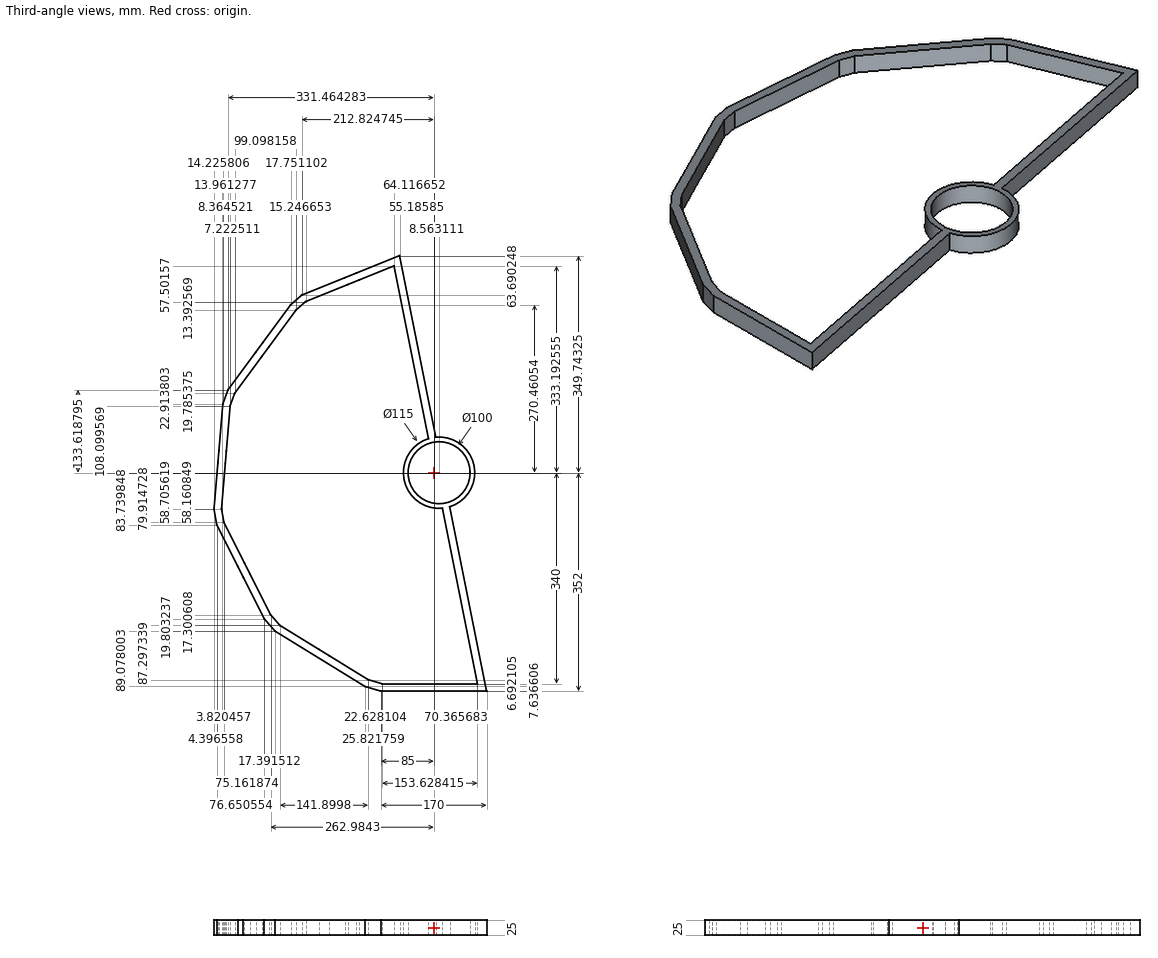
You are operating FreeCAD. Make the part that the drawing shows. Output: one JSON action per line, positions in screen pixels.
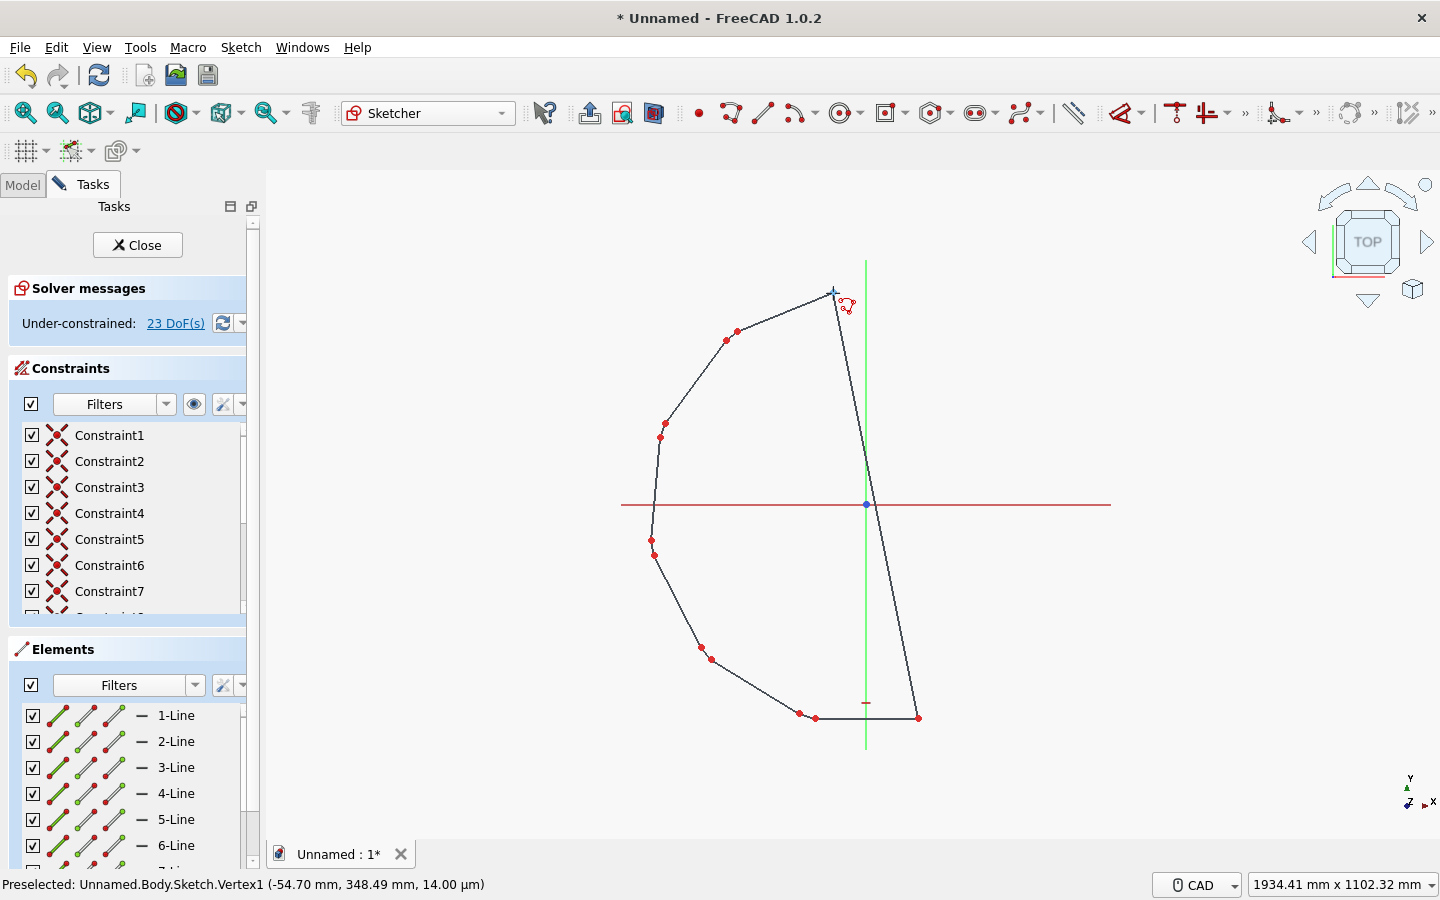
{"action": "scroll", "coordinate": [827, 302], "scroll_direction": "up", "scroll_amount": 4}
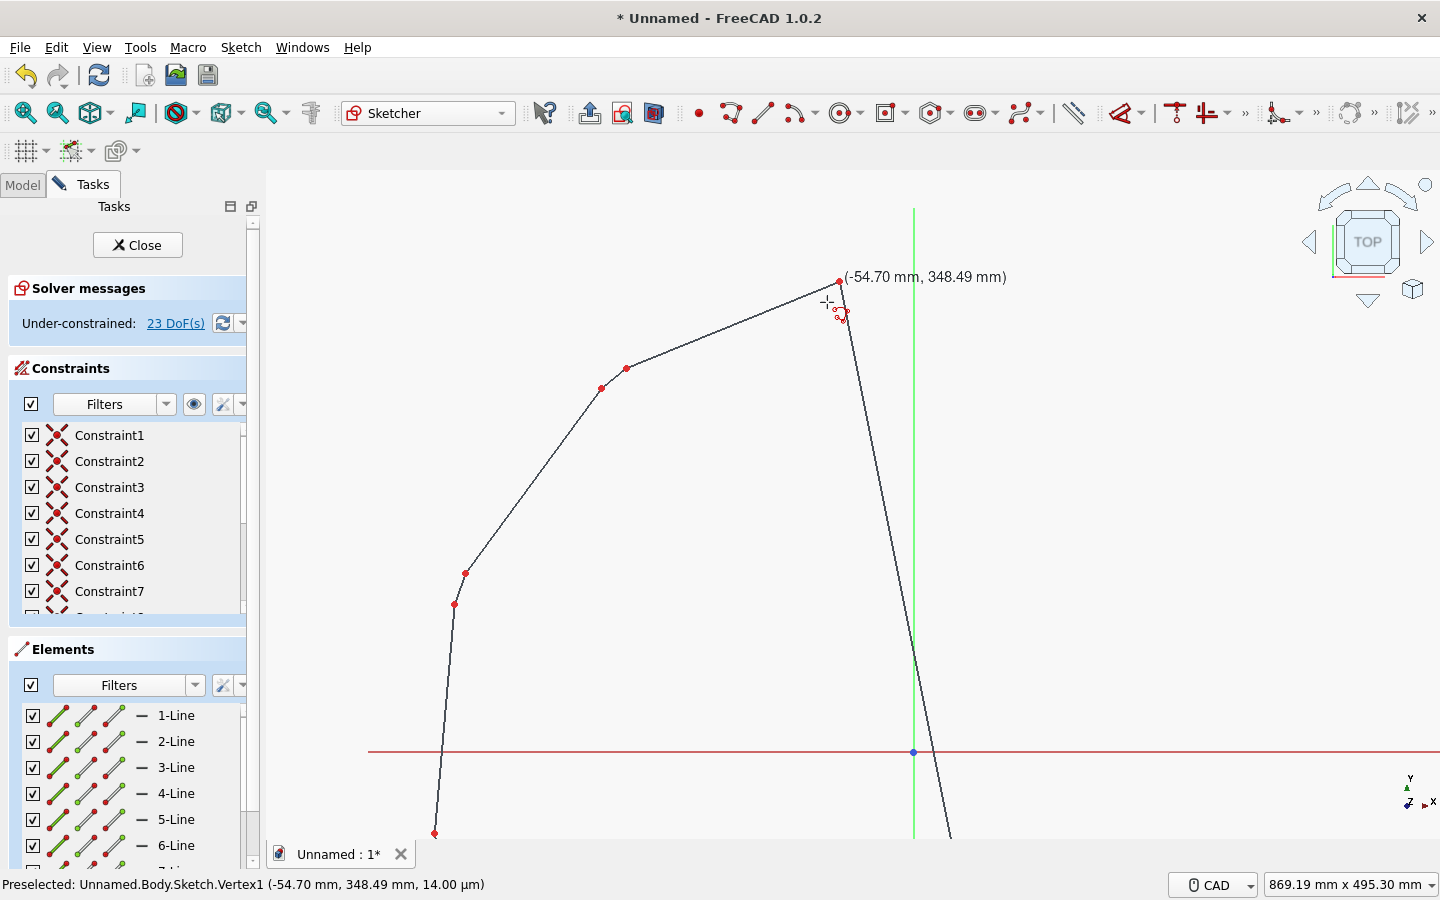
{"action": "left_click", "coordinate": [827, 302]}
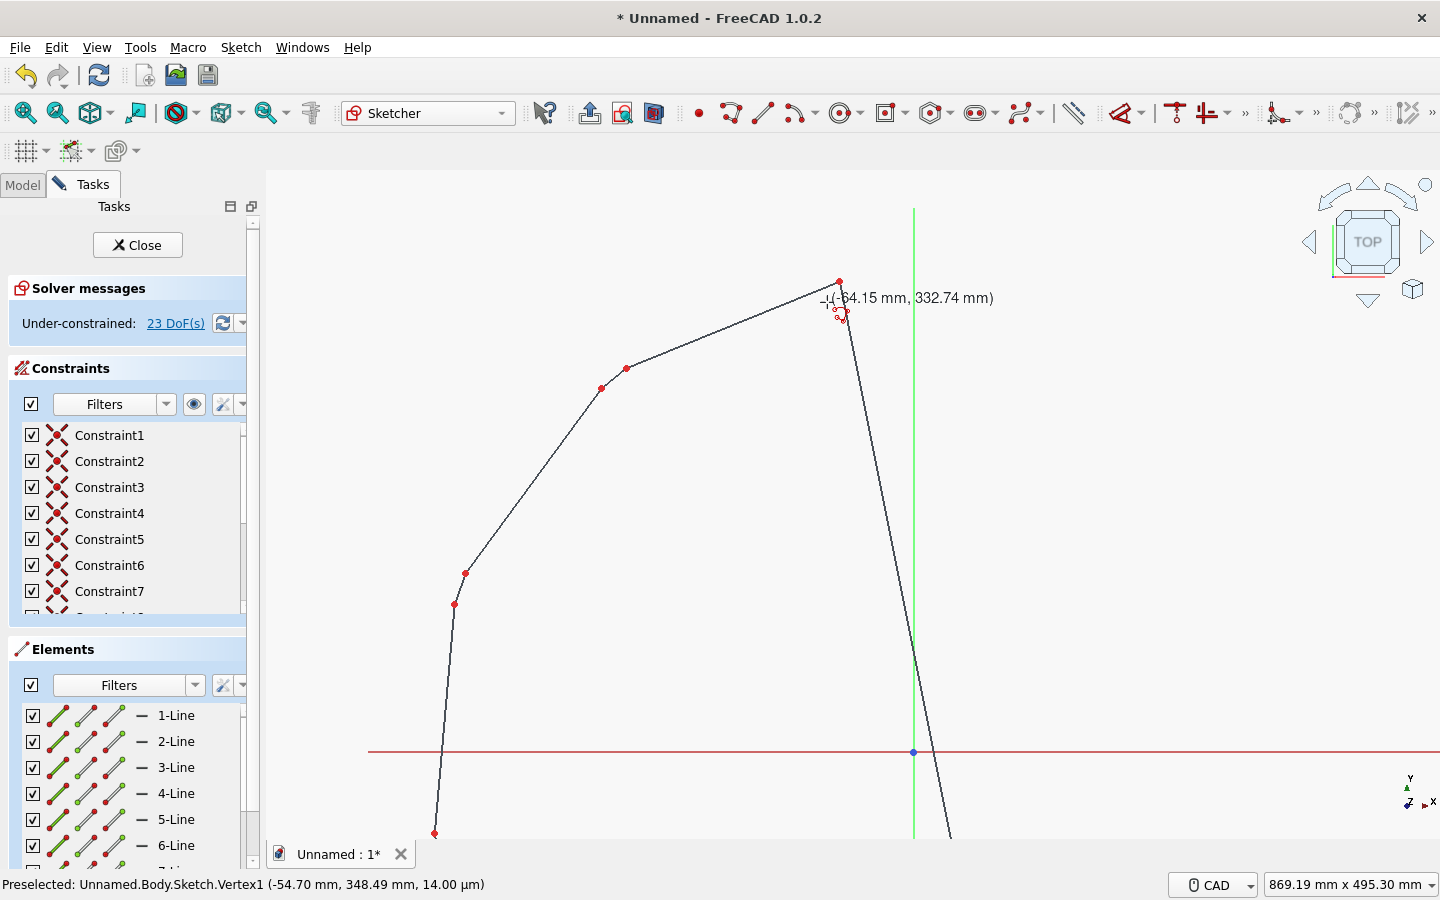
{"action": "scroll", "coordinate": [827, 301], "scroll_direction": "down", "scroll_amount": 4}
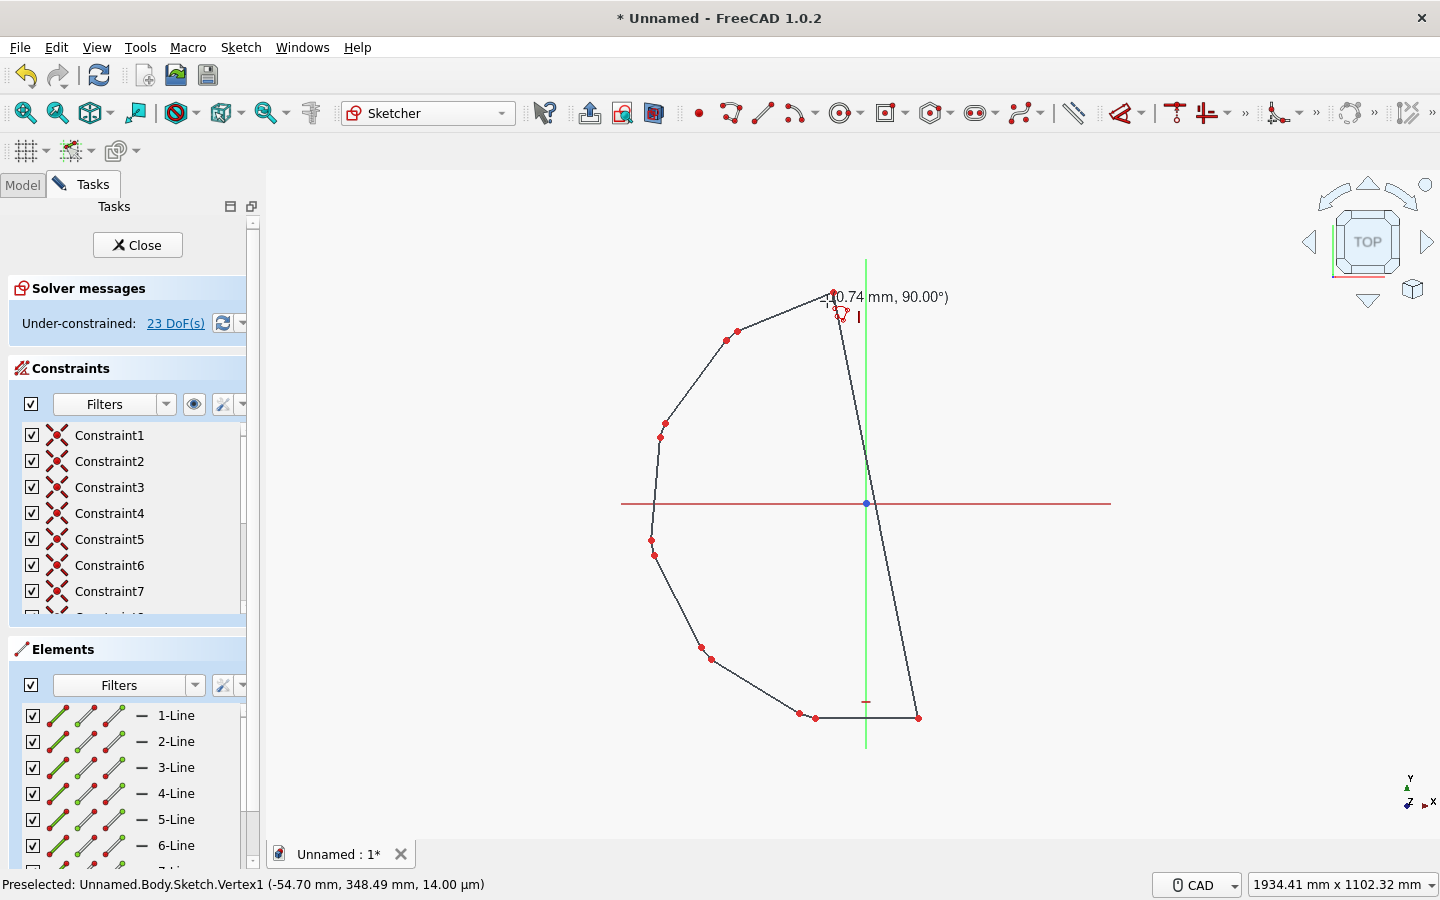
{"action": "scroll", "coordinate": [909, 710], "scroll_direction": "up", "scroll_amount": 4}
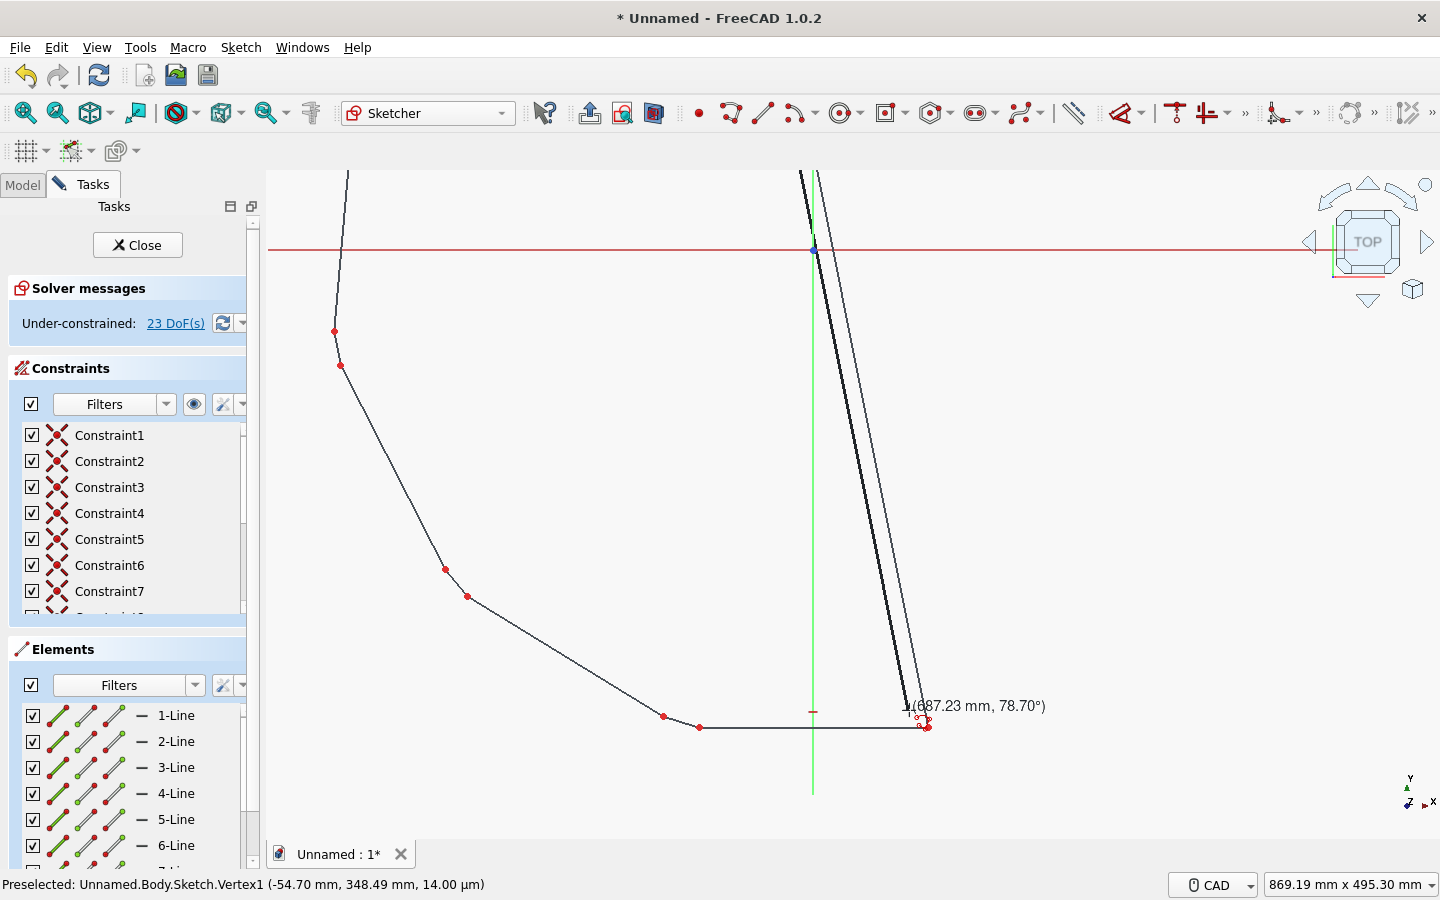
{"action": "left_click", "coordinate": [908, 710]}
{"action": "left_click", "coordinate": [701, 710]}
{"action": "left_click", "coordinate": [670, 701]}
{"action": "left_click", "coordinate": [478, 583]}
{"action": "left_click", "coordinate": [458, 559]}
{"action": "left_click", "coordinate": [356, 358]}
{"action": "left_click", "coordinate": [351, 329]}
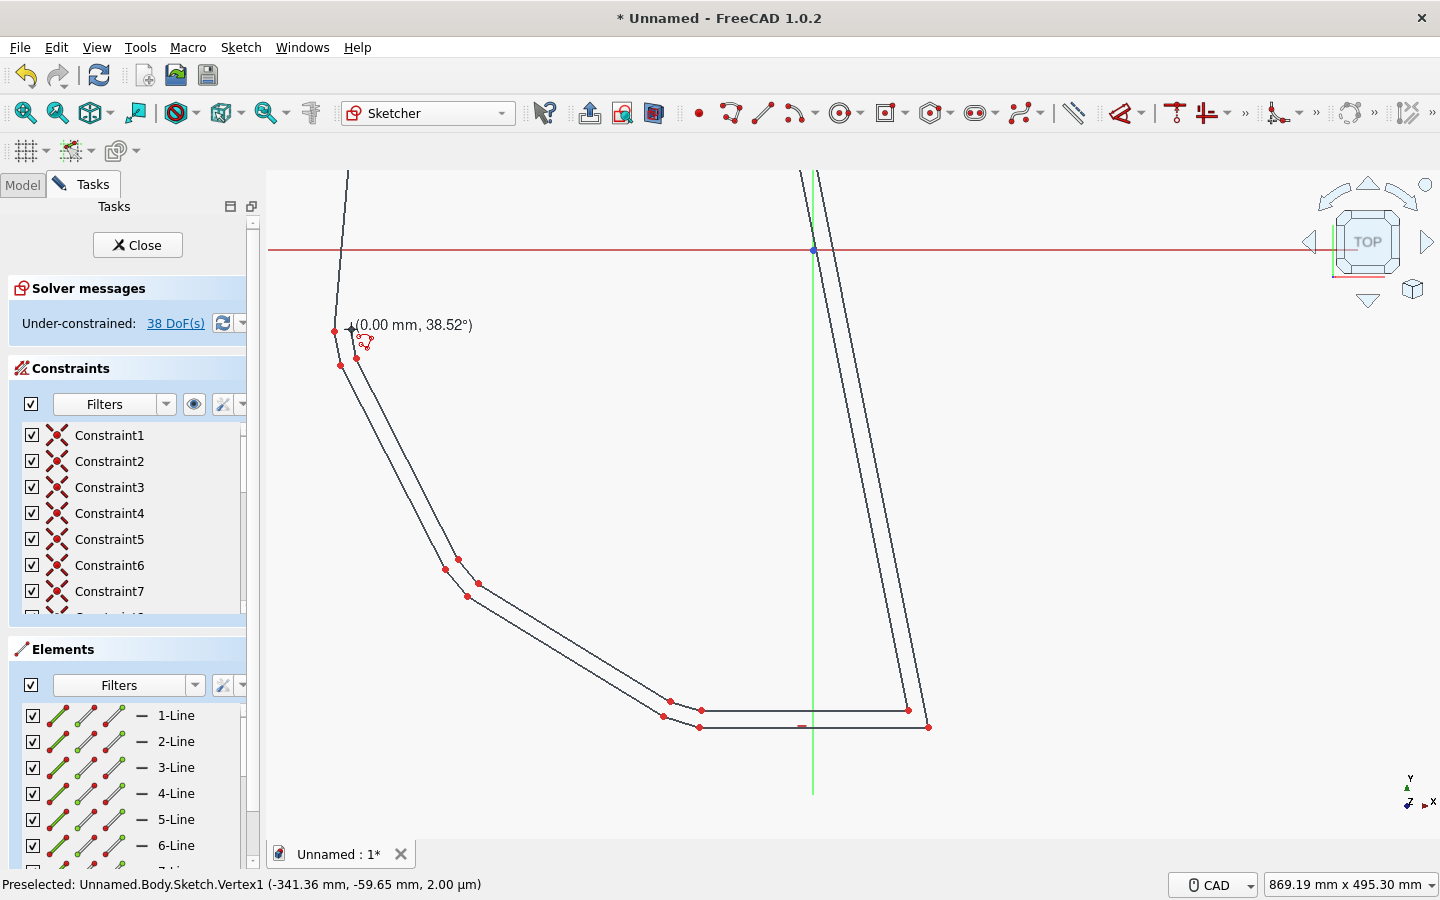
{"action": "scroll", "coordinate": [909, 711], "scroll_direction": "down", "scroll_amount": 4}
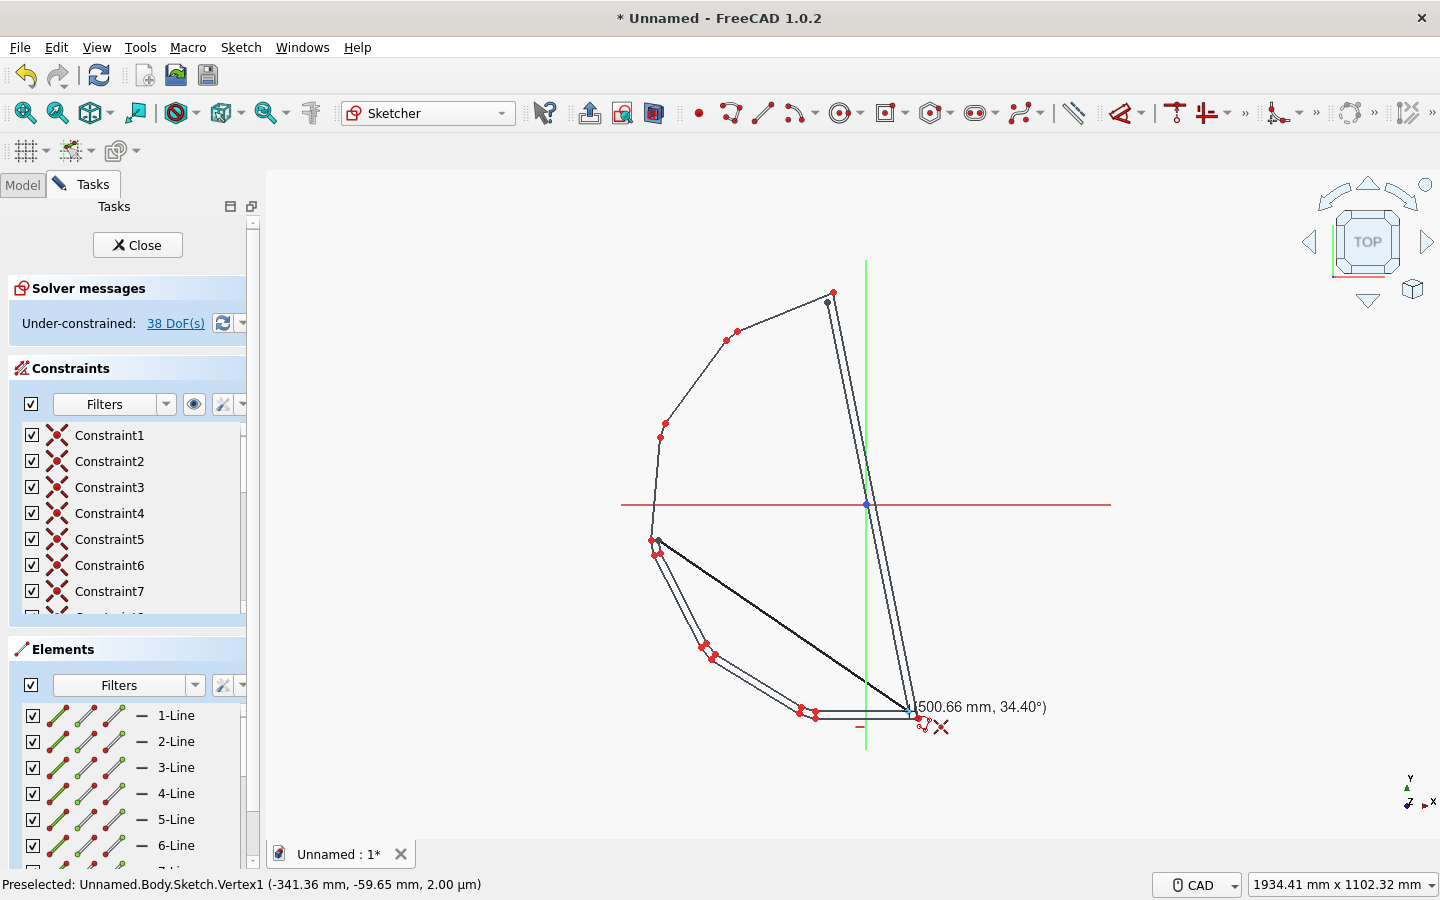
{"action": "scroll", "coordinate": [667, 439], "scroll_direction": "up", "scroll_amount": 4}